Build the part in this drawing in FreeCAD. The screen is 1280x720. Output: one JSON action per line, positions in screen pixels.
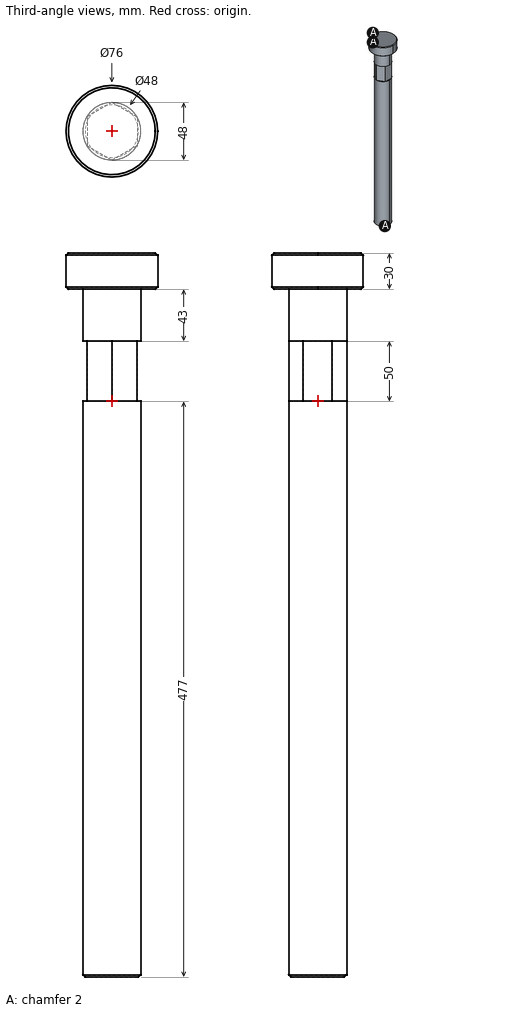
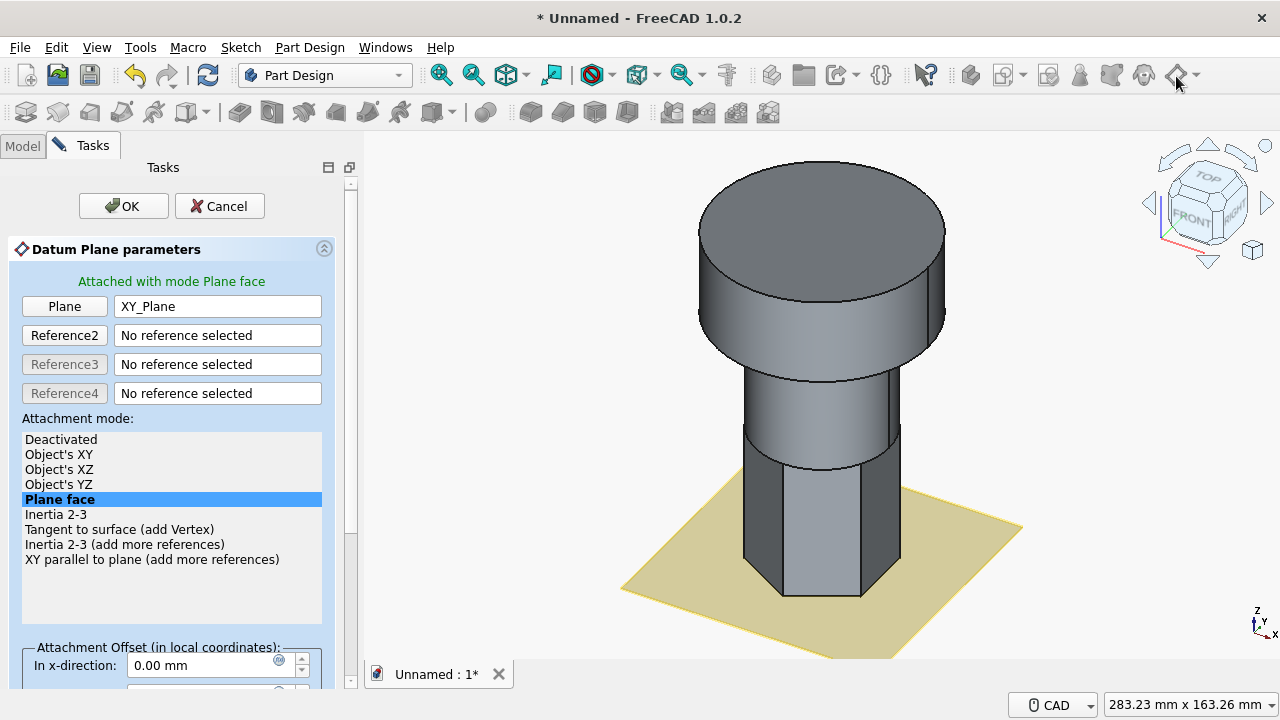
{"action": "scroll", "coordinate": [351, 432], "scroll_direction": "down", "scroll_amount": 2}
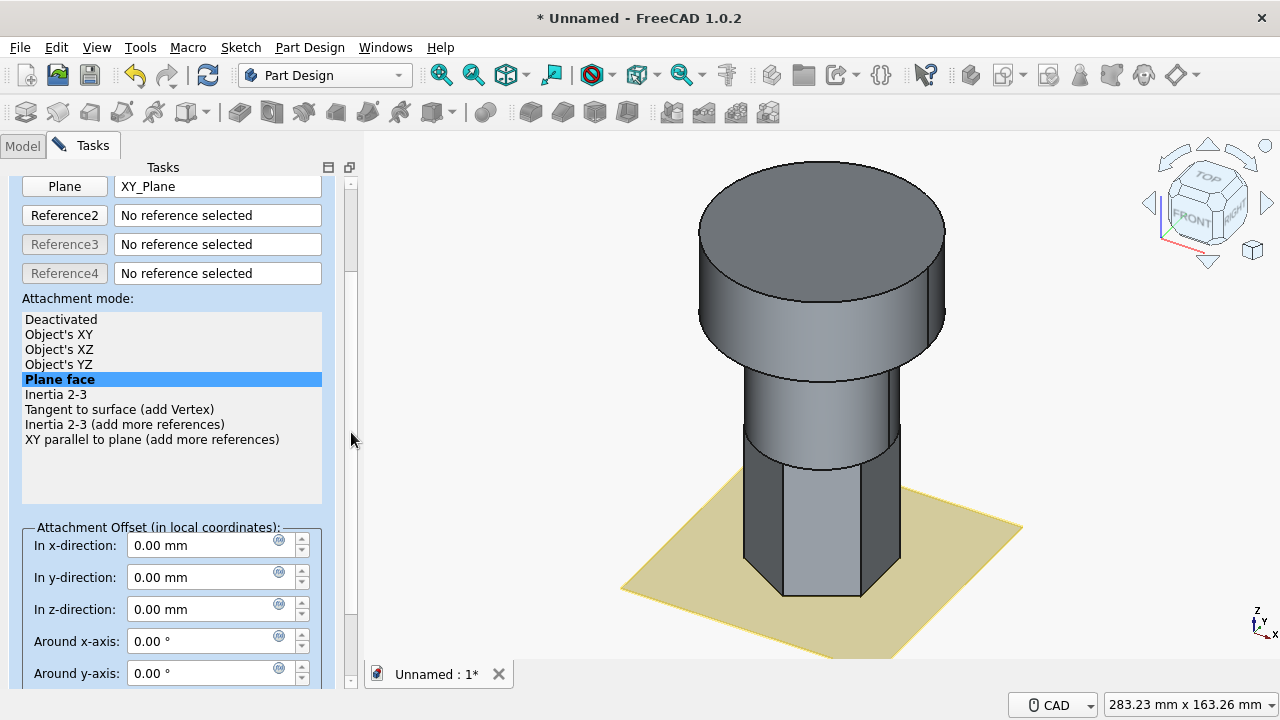
{"action": "triple_click", "coordinate": [210, 609]}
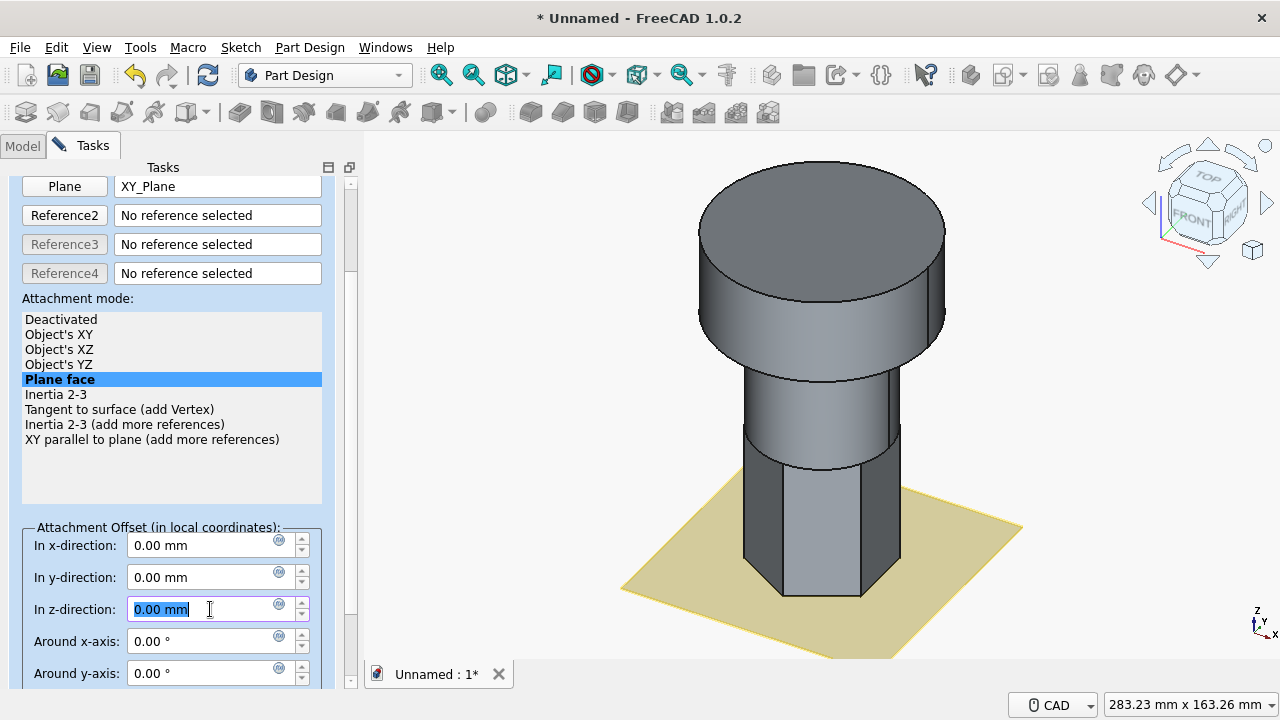
{"action": "type", "text": "-477"}
{"action": "key", "text": "Tab"}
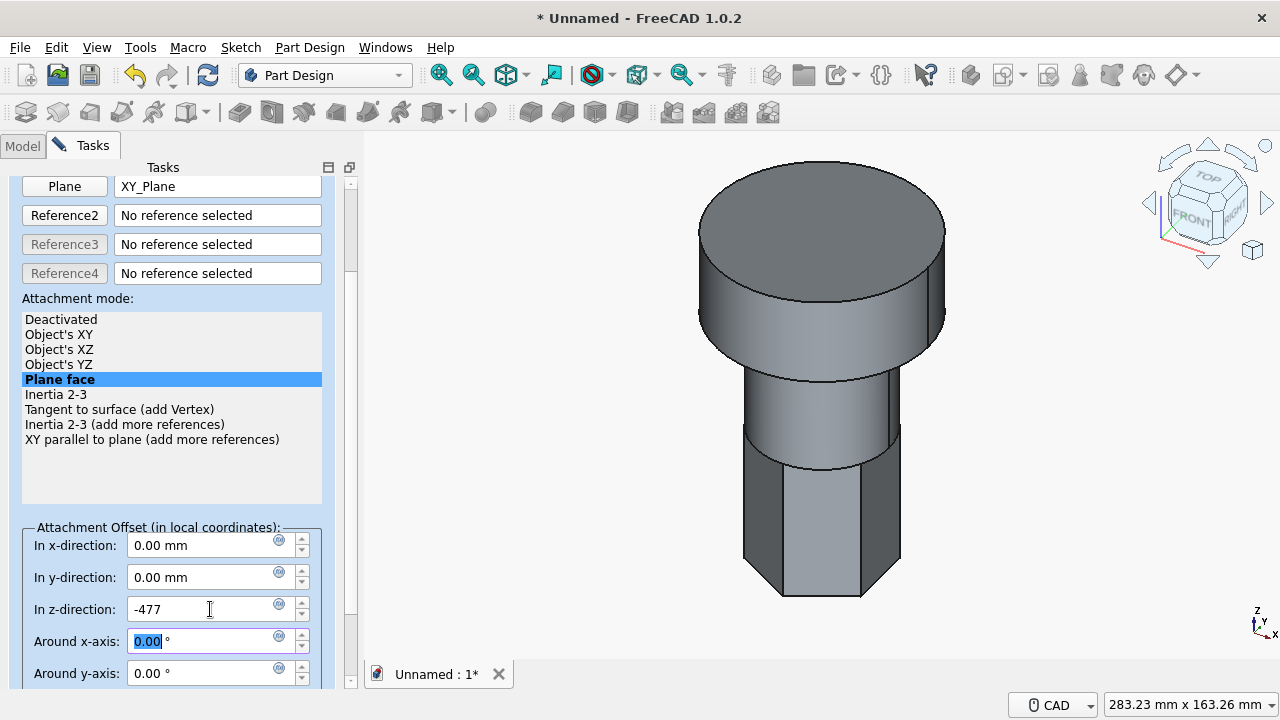
{"action": "scroll", "coordinate": [351, 432], "scroll_direction": "up", "scroll_amount": 3}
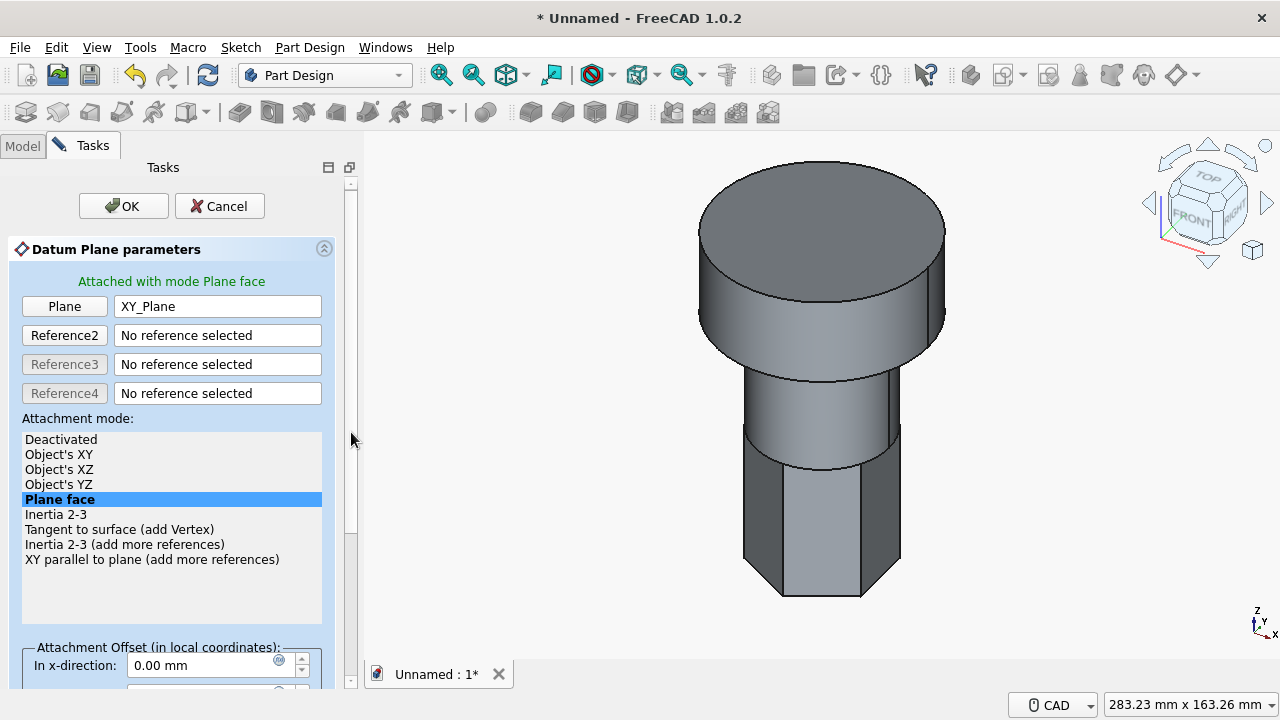
{"action": "left_click", "coordinate": [124, 206]}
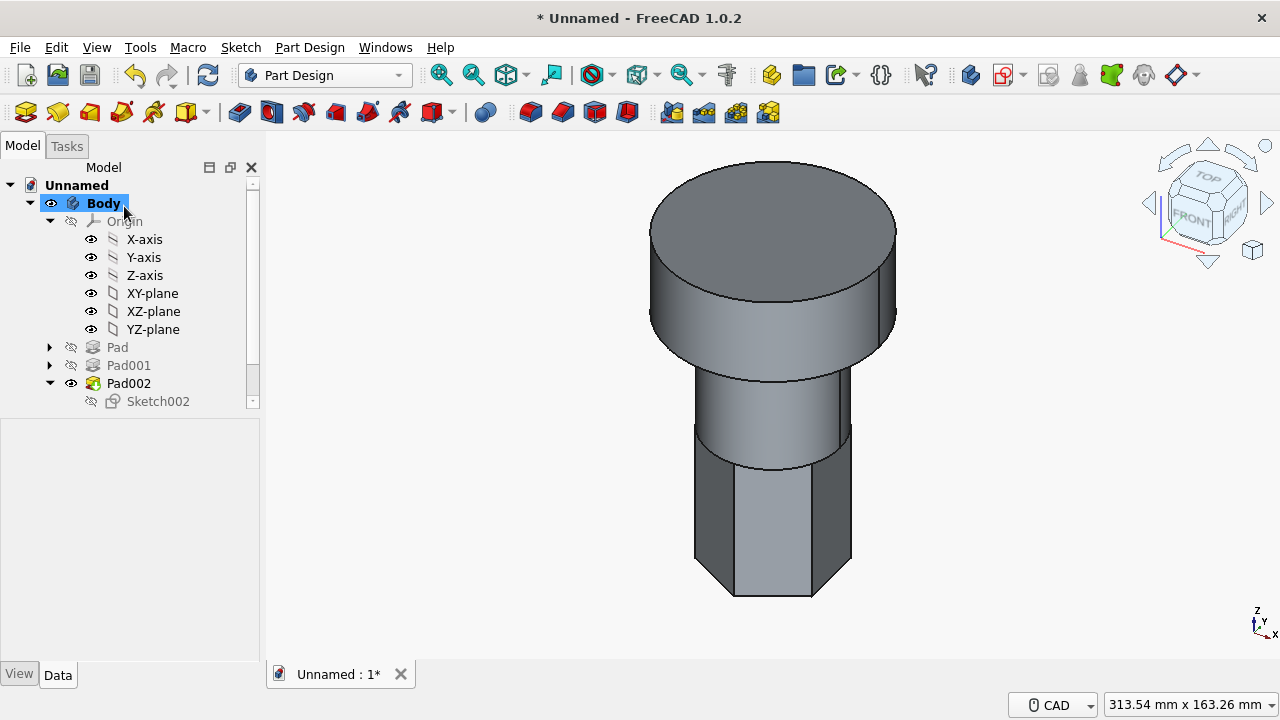
{"action": "scroll", "coordinate": [100, 289], "scroll_direction": "down", "scroll_amount": 3}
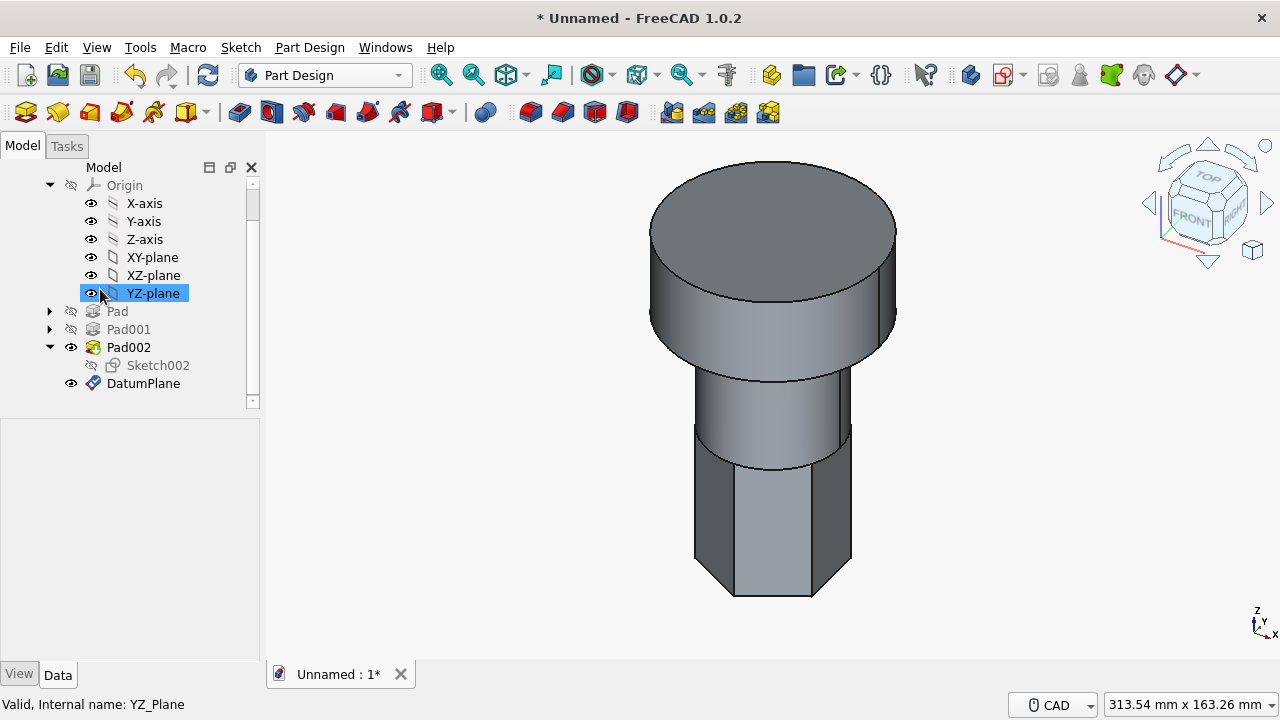
{"action": "left_click", "coordinate": [116, 383]}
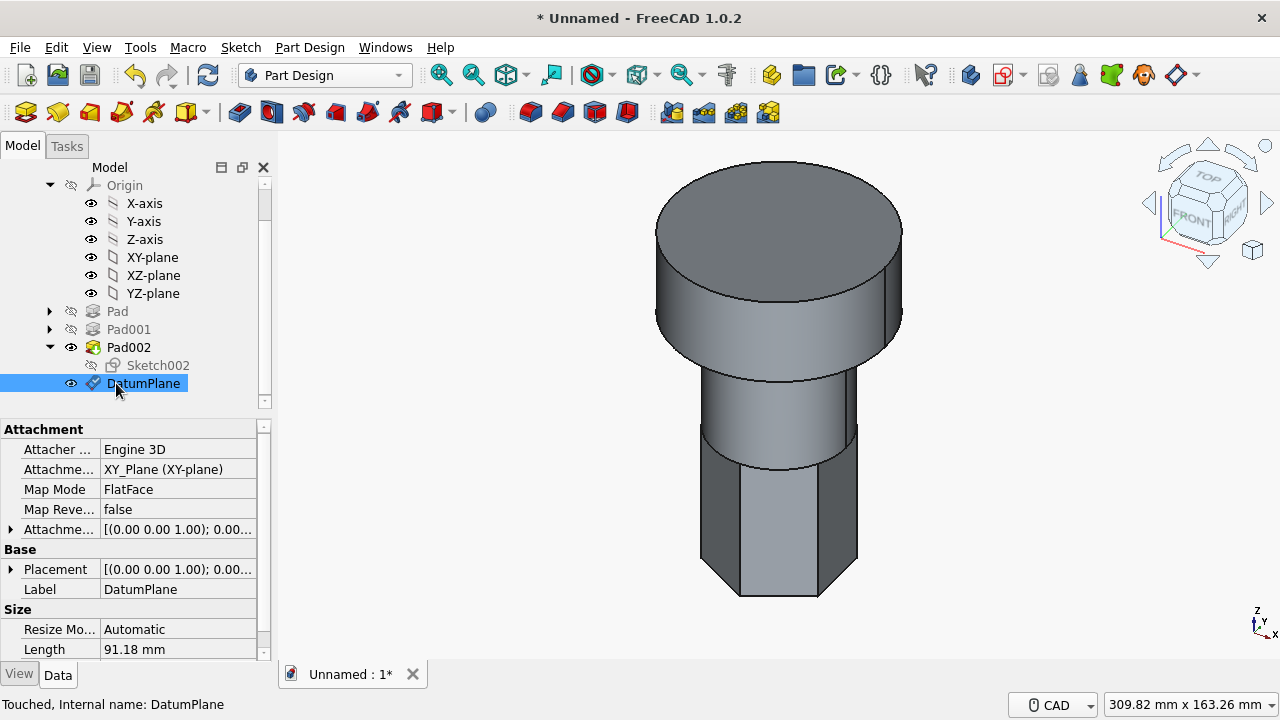
{"action": "left_click", "coordinate": [1004, 76]}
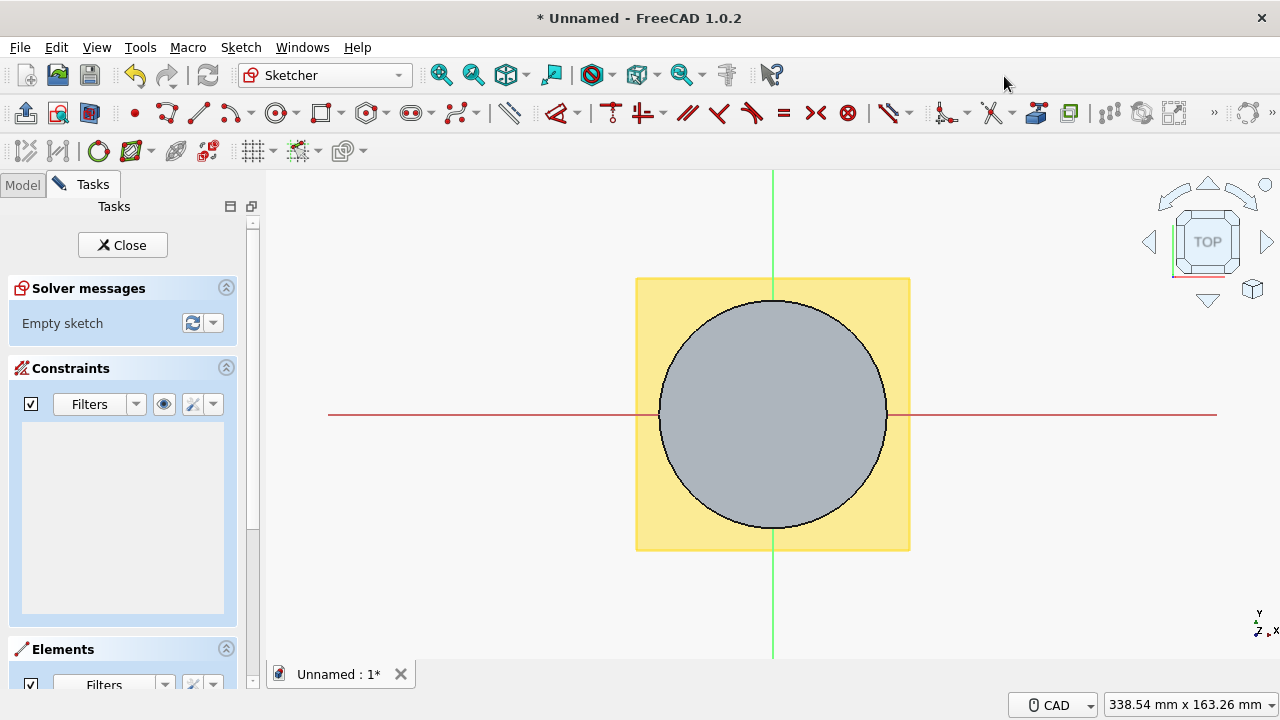
{"action": "left_click", "coordinate": [90, 114]}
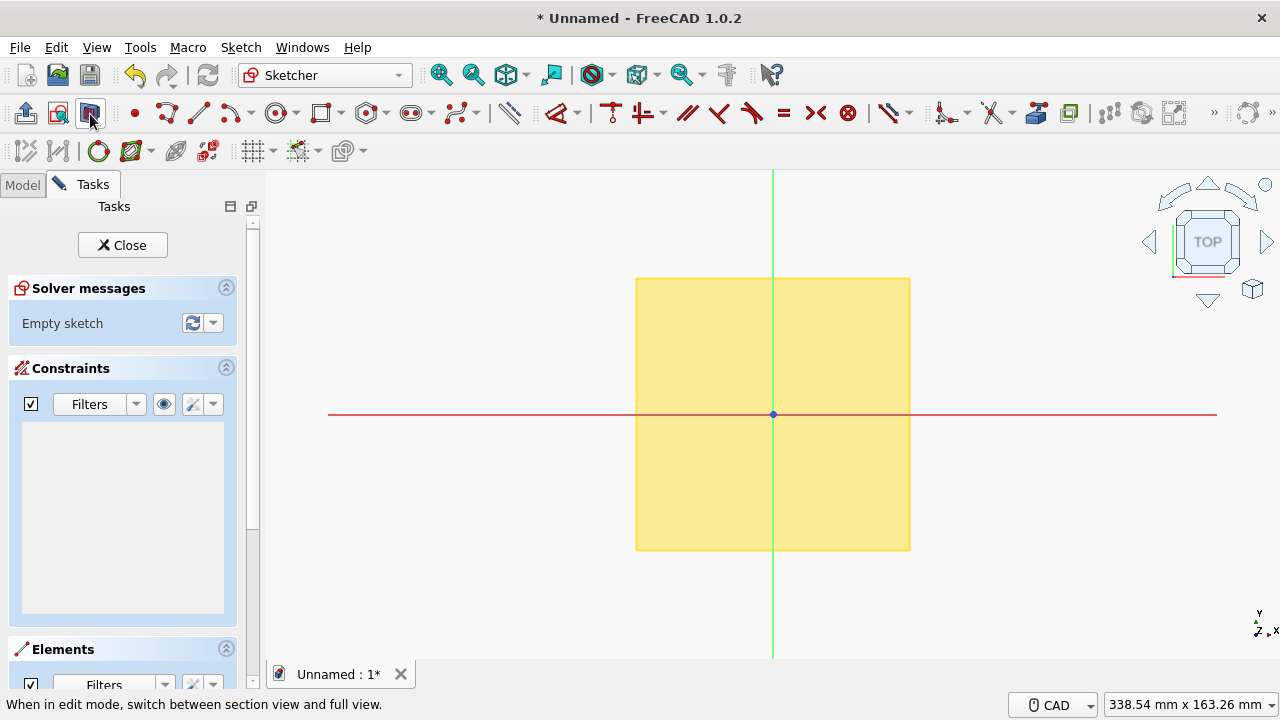
{"action": "scroll", "coordinate": [829, 414], "scroll_direction": "up", "scroll_amount": 4}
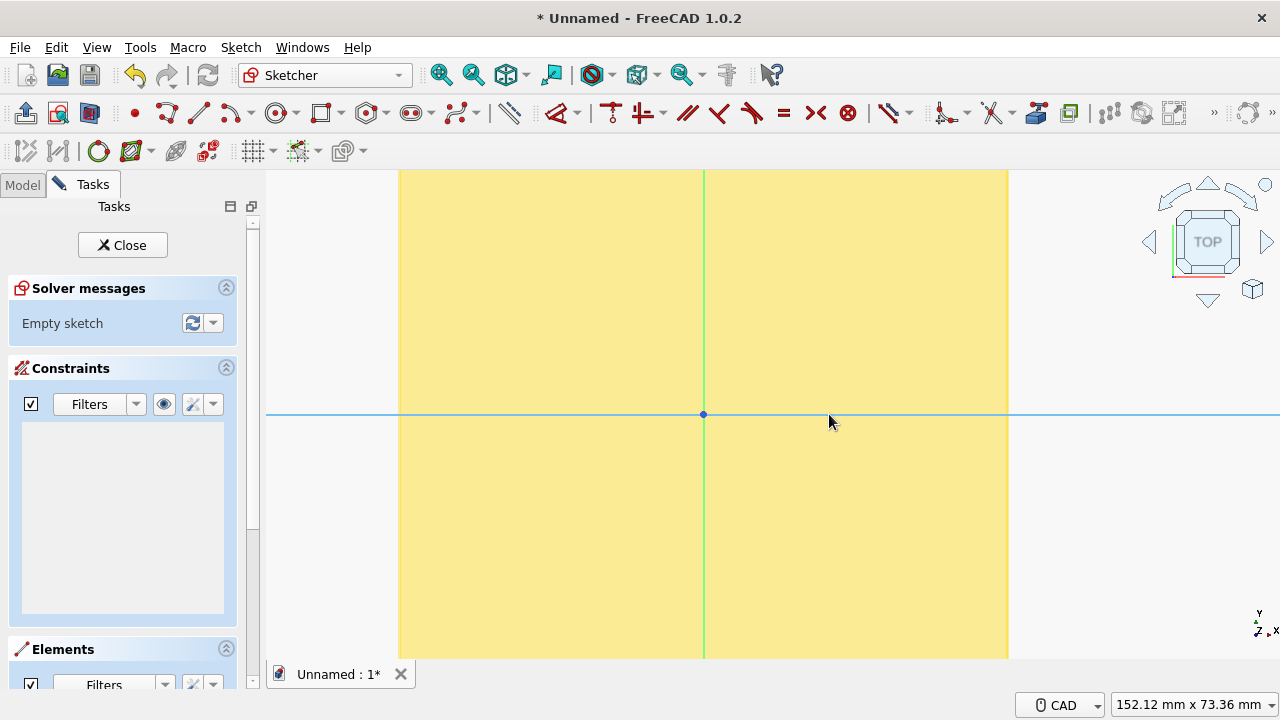
{"action": "left_click", "coordinate": [276, 114]}